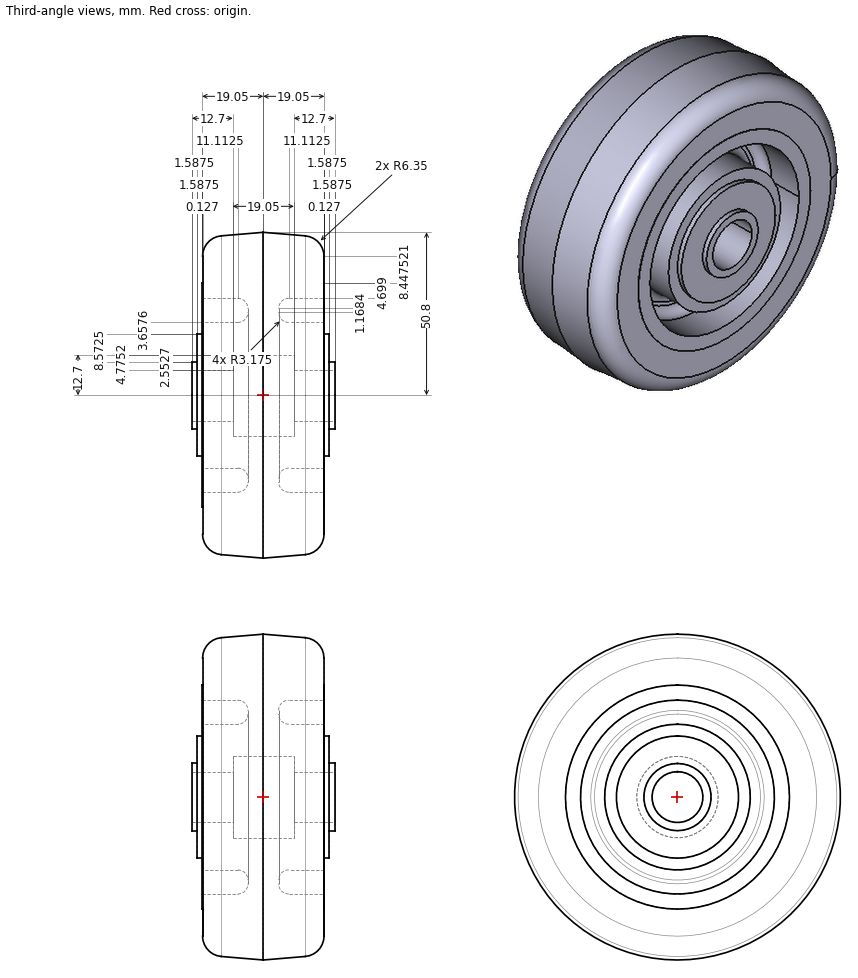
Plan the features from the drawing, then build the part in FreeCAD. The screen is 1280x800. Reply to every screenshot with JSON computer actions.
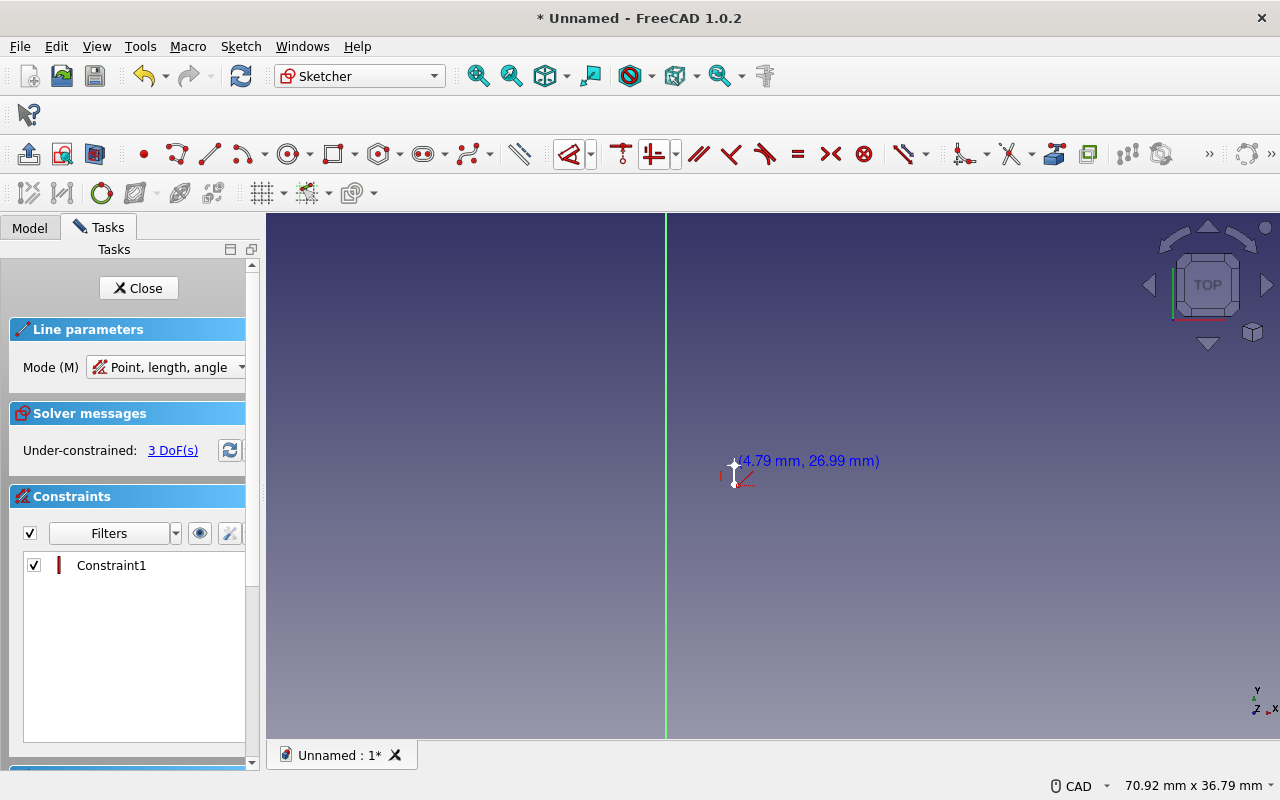
{"action": "left_click", "coordinate": [177, 154]}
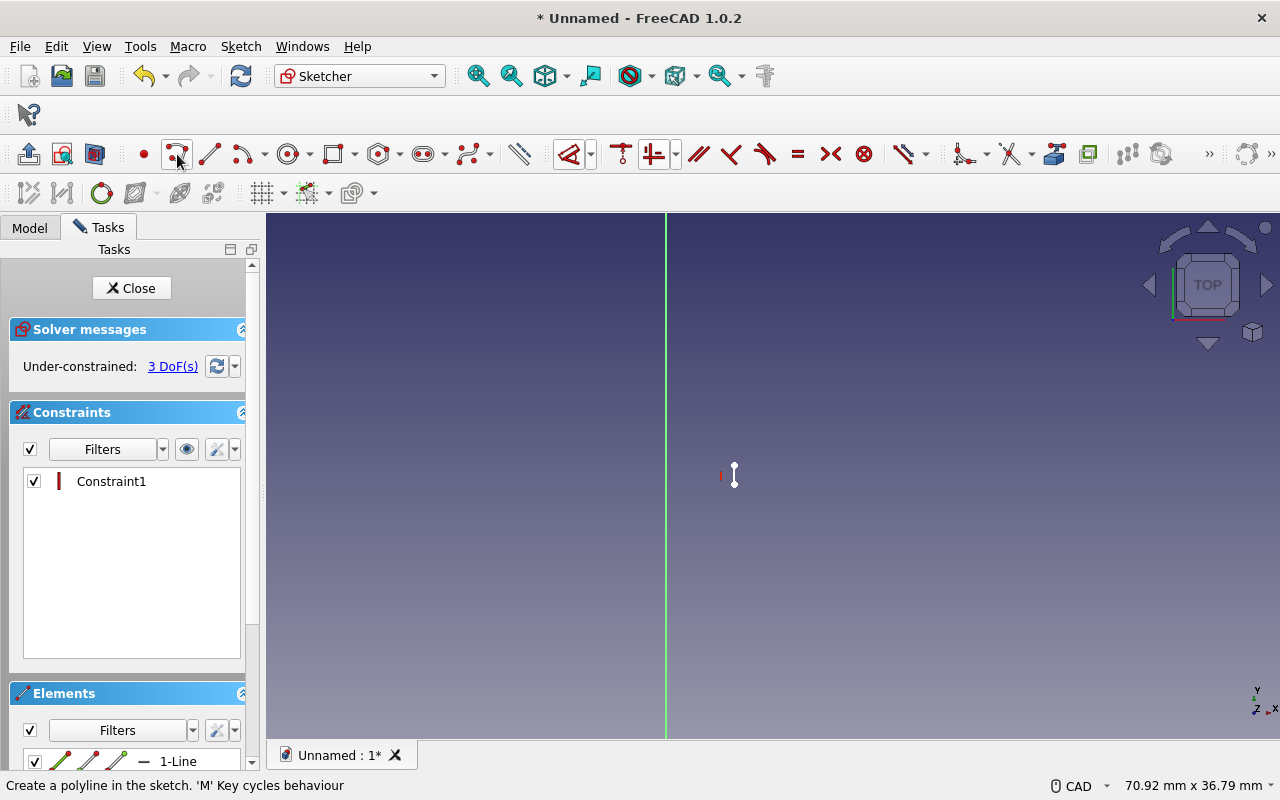
{"action": "left_click", "coordinate": [779, 420]}
{"action": "left_click", "coordinate": [938, 420]}
{"action": "left_click", "coordinate": [938, 353]}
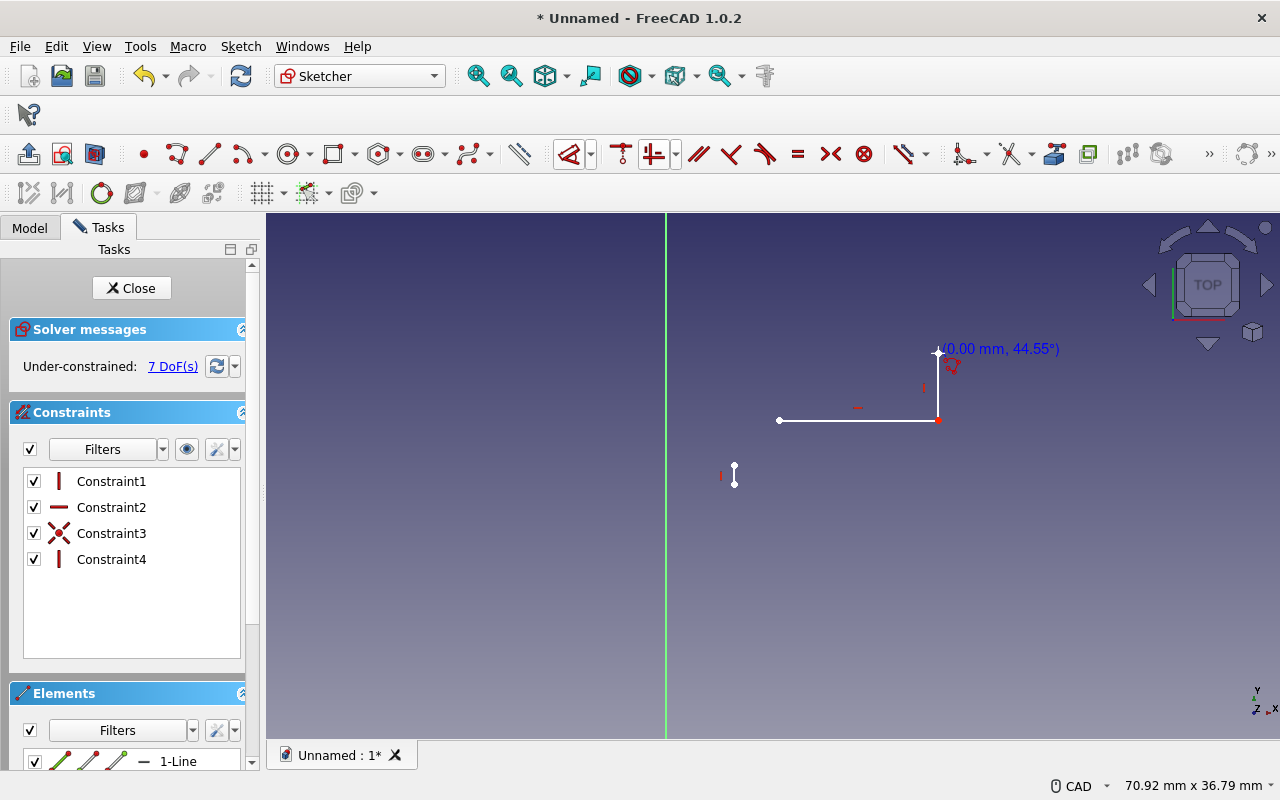
{"action": "scroll", "coordinate": [936, 353], "scroll_direction": "up", "scroll_amount": 11}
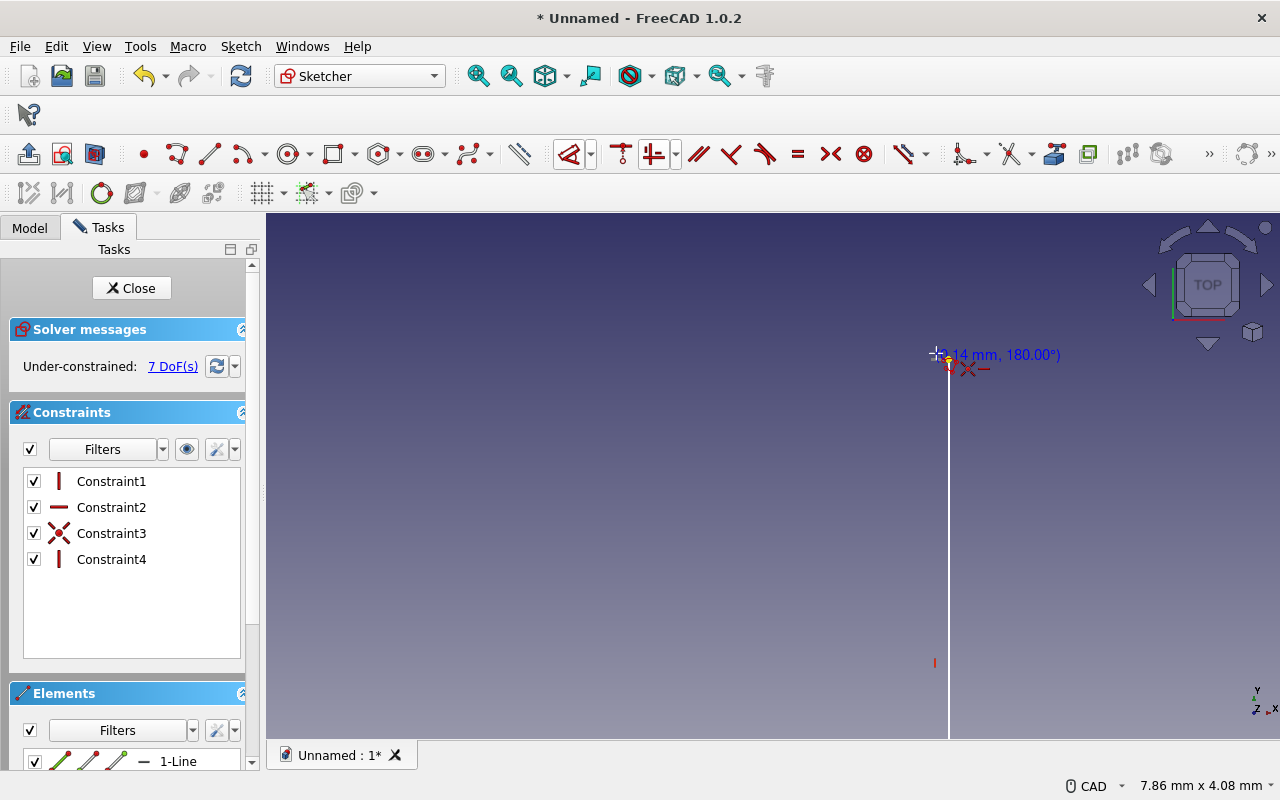
{"action": "left_click", "coordinate": [932, 351]}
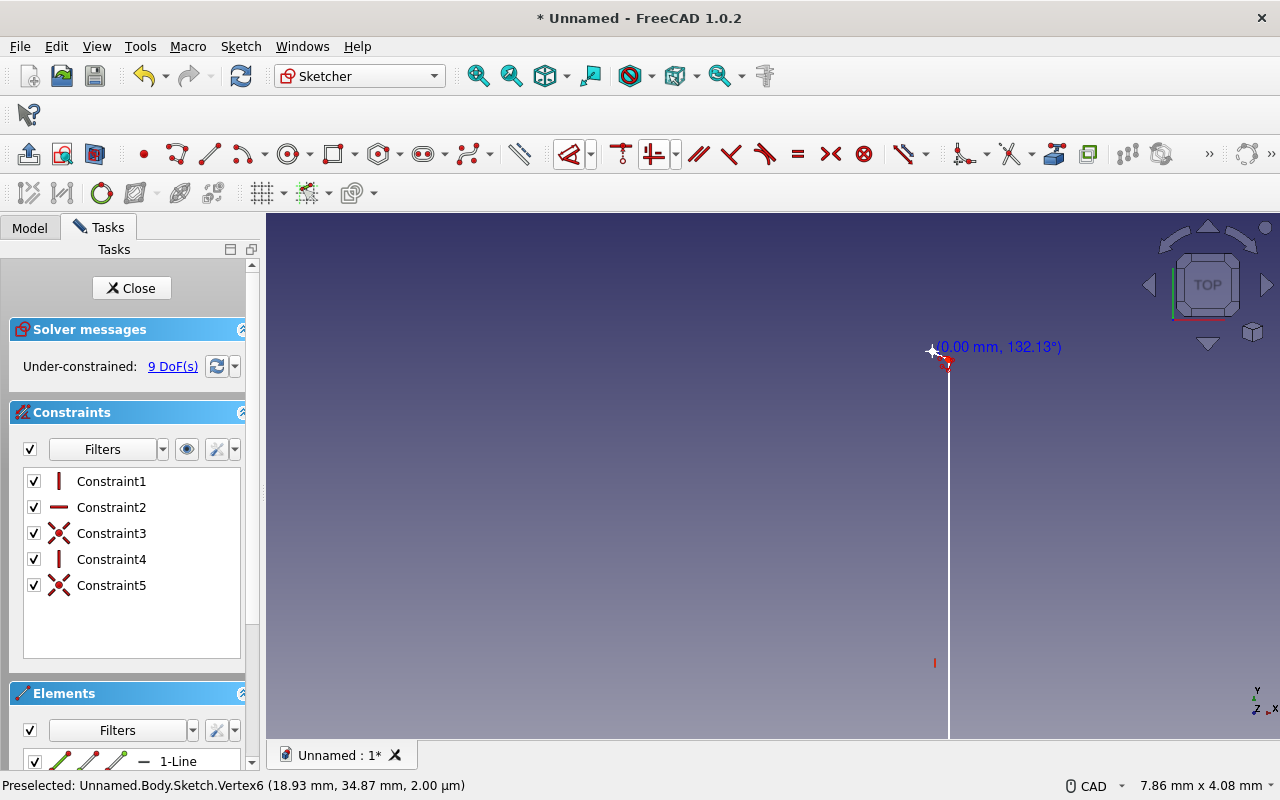
{"action": "scroll", "coordinate": [821, 418], "scroll_direction": "down", "scroll_amount": 15}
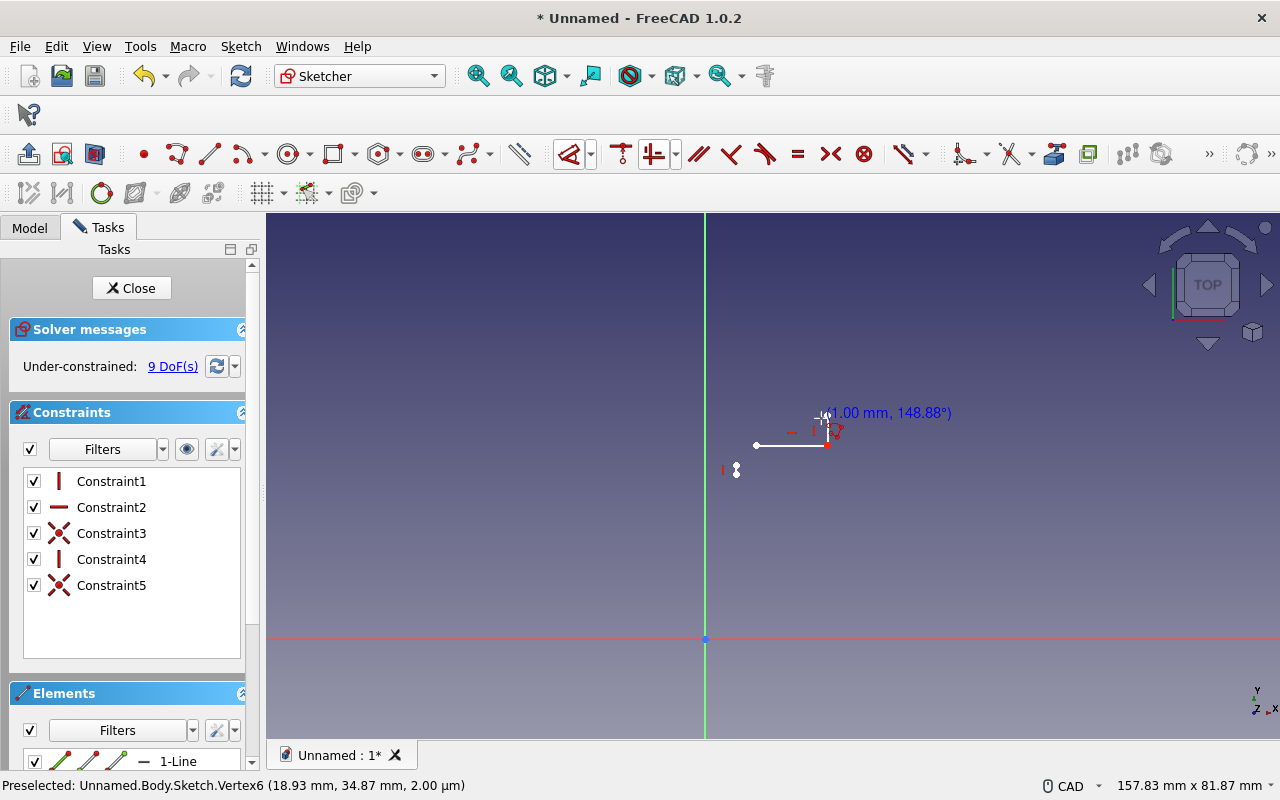
{"action": "left_click", "coordinate": [827, 361]}
{"action": "right_click", "coordinate": [827, 361]}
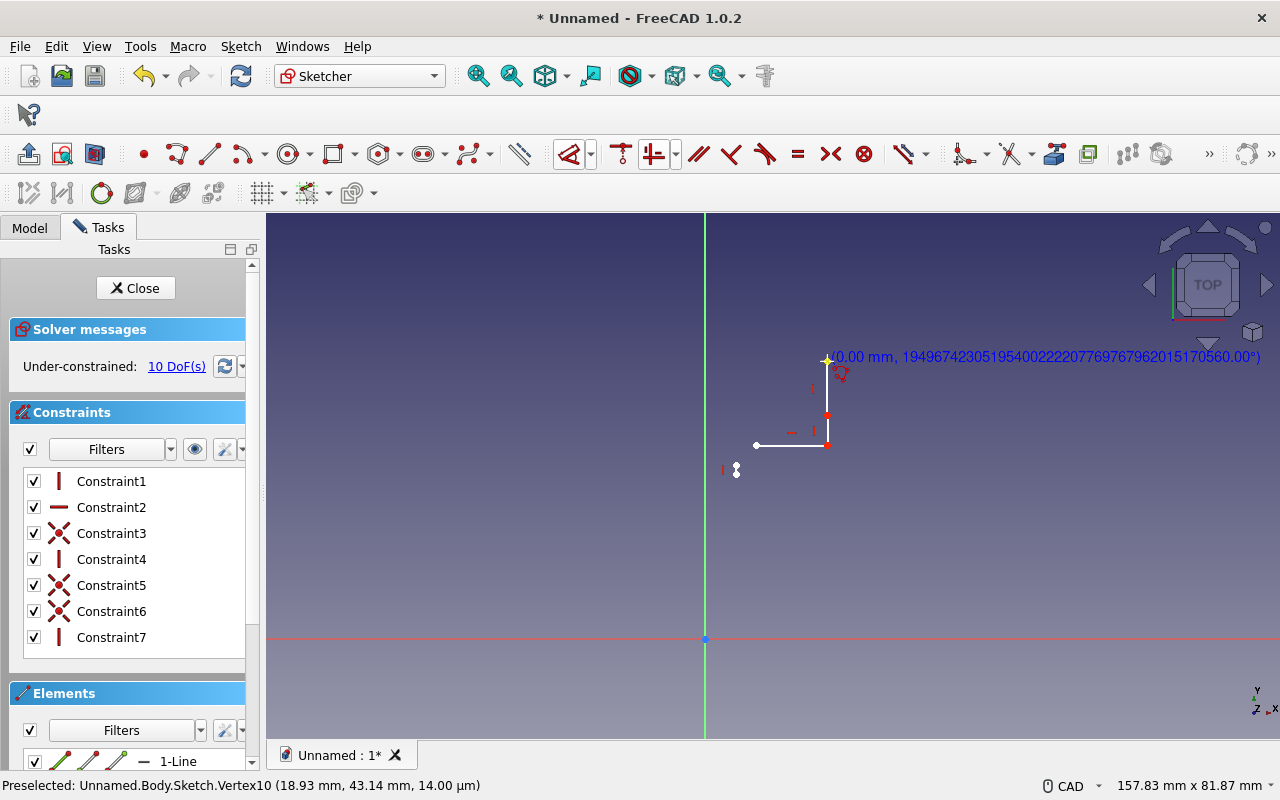
{"action": "left_click", "coordinate": [790, 320]}
{"action": "left_click", "coordinate": [705, 313]}
{"action": "left_click", "coordinate": [621, 320]}
{"action": "right_click", "coordinate": [621, 320]}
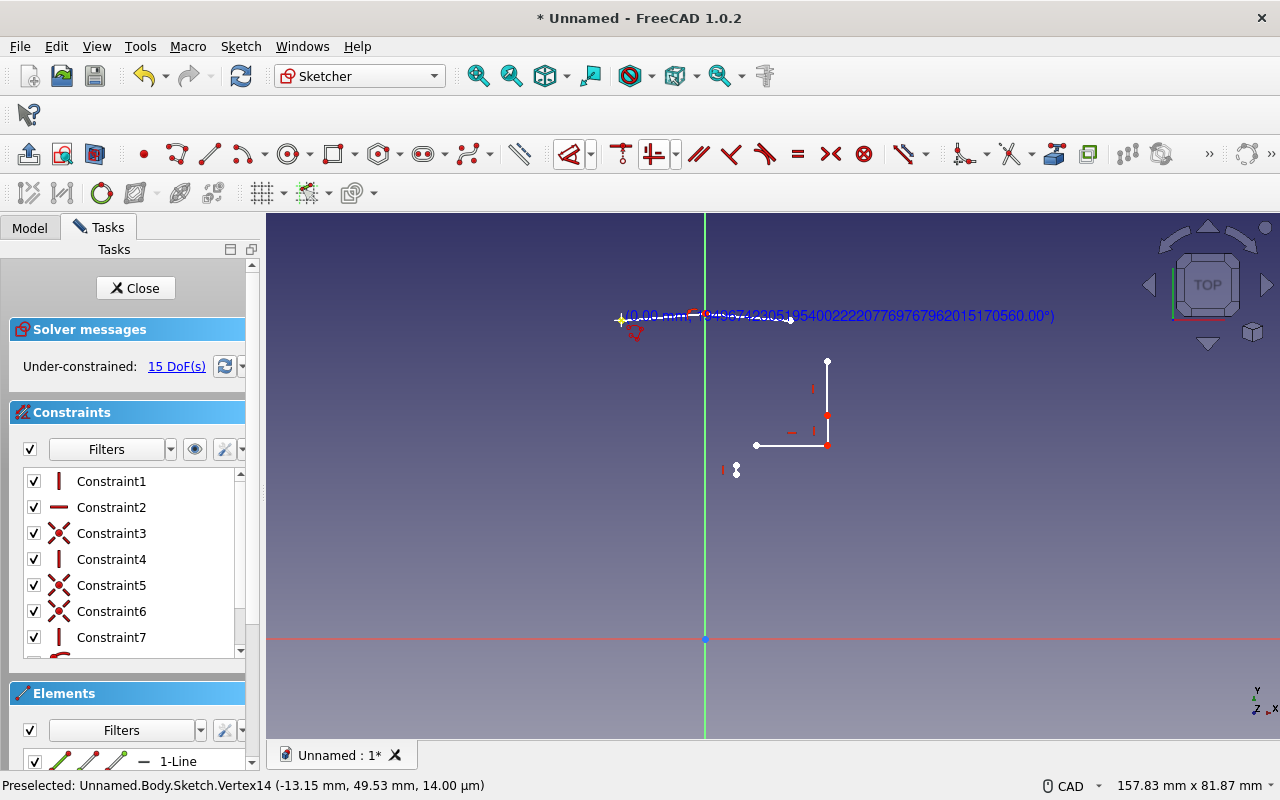
{"action": "left_click", "coordinate": [584, 361]}
{"action": "left_click", "coordinate": [584, 415]}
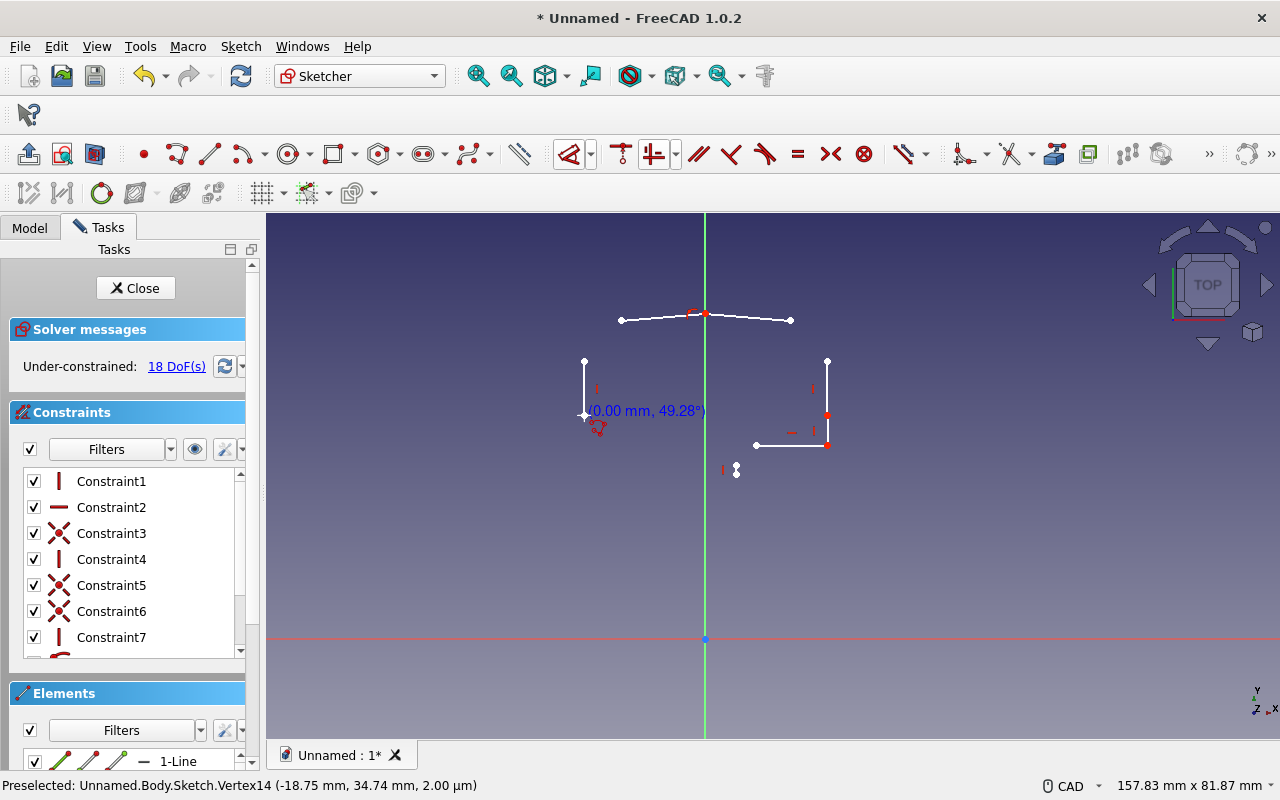
{"action": "scroll", "coordinate": [583, 415], "scroll_direction": "up", "scroll_amount": 15}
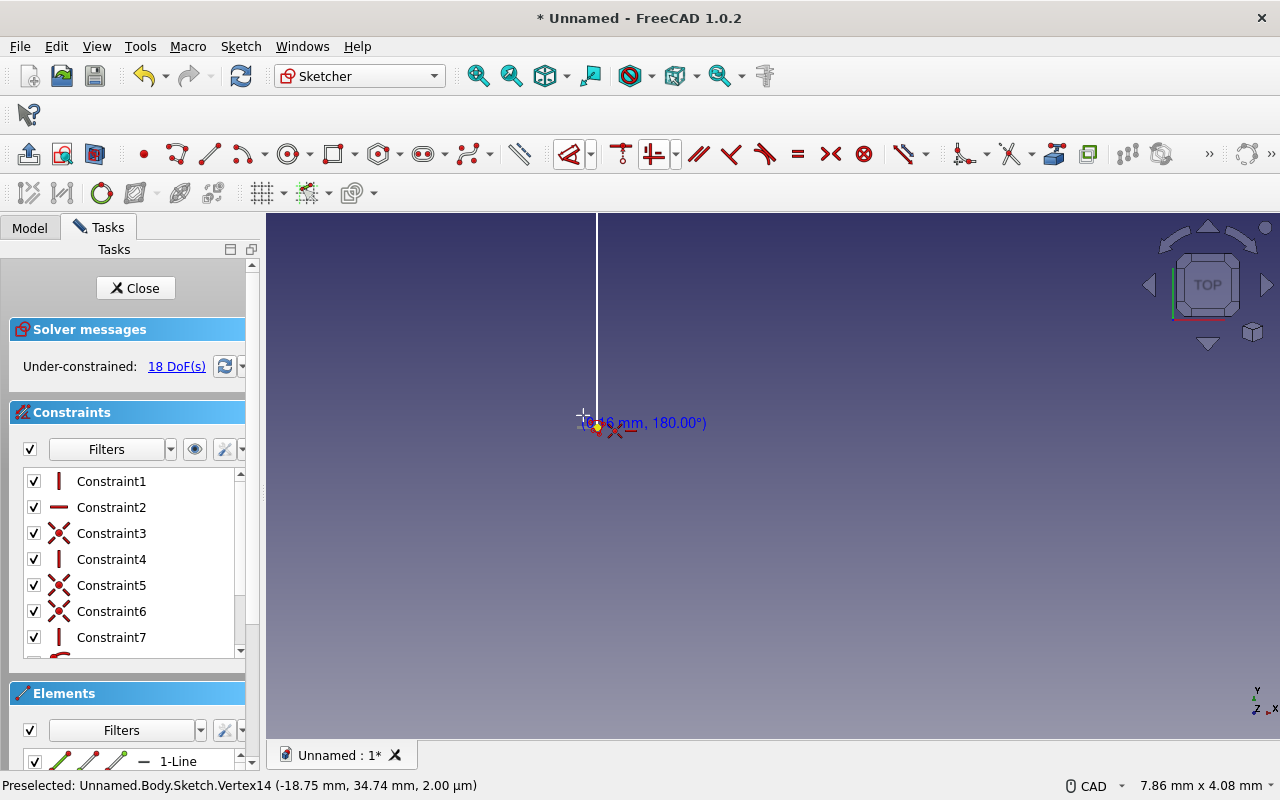
{"action": "left_click", "coordinate": [578, 408]}